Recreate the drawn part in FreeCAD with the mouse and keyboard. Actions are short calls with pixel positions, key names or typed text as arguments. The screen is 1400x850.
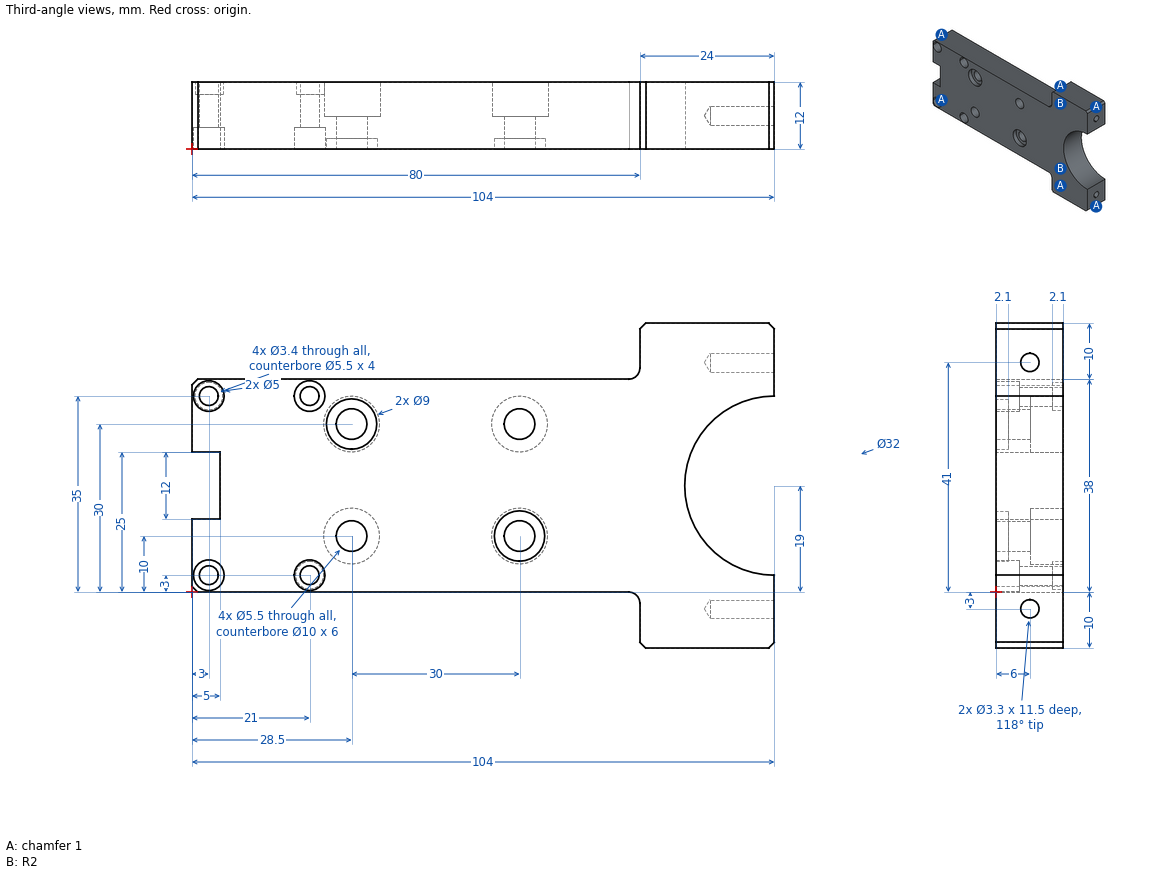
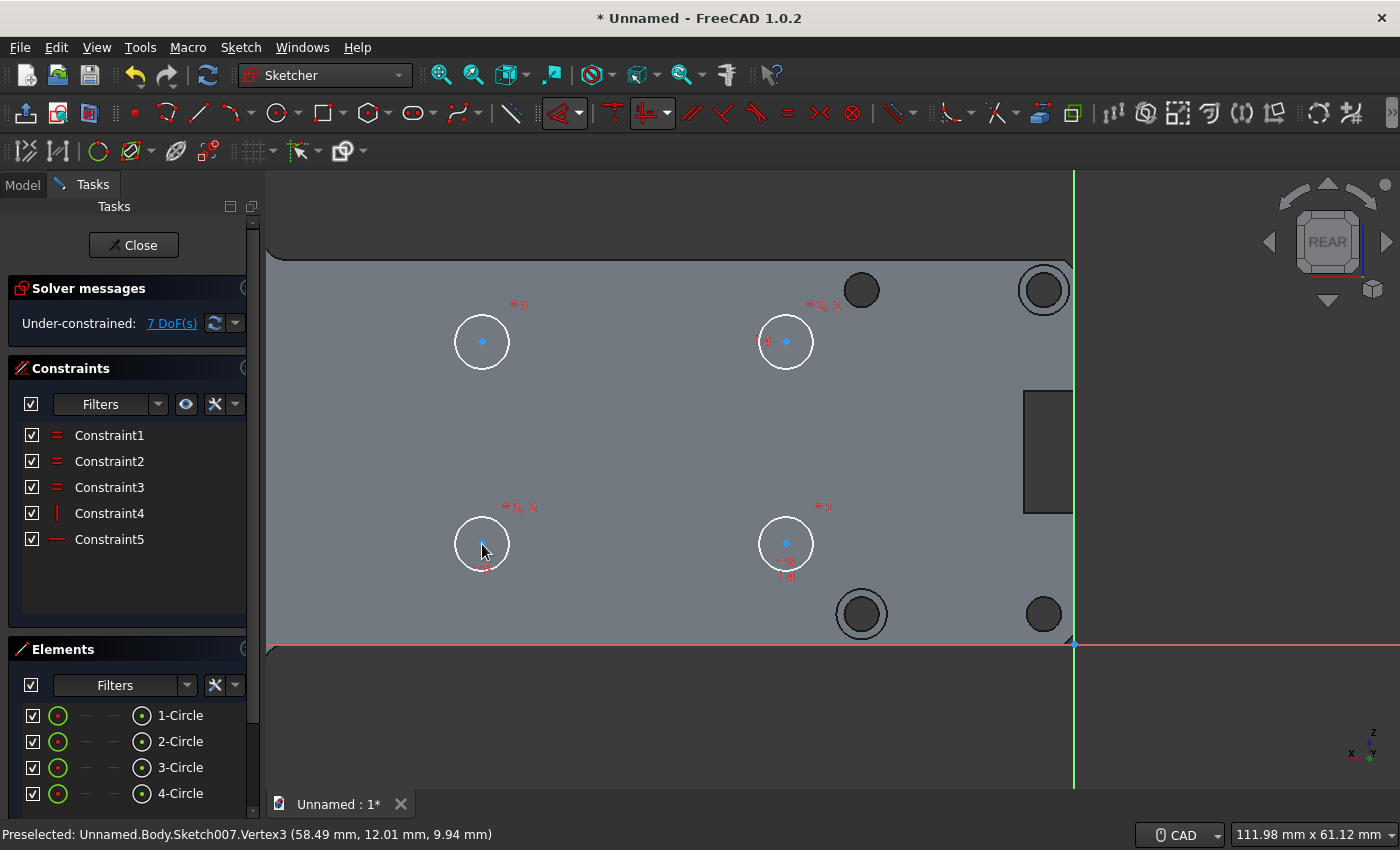
click(482, 544)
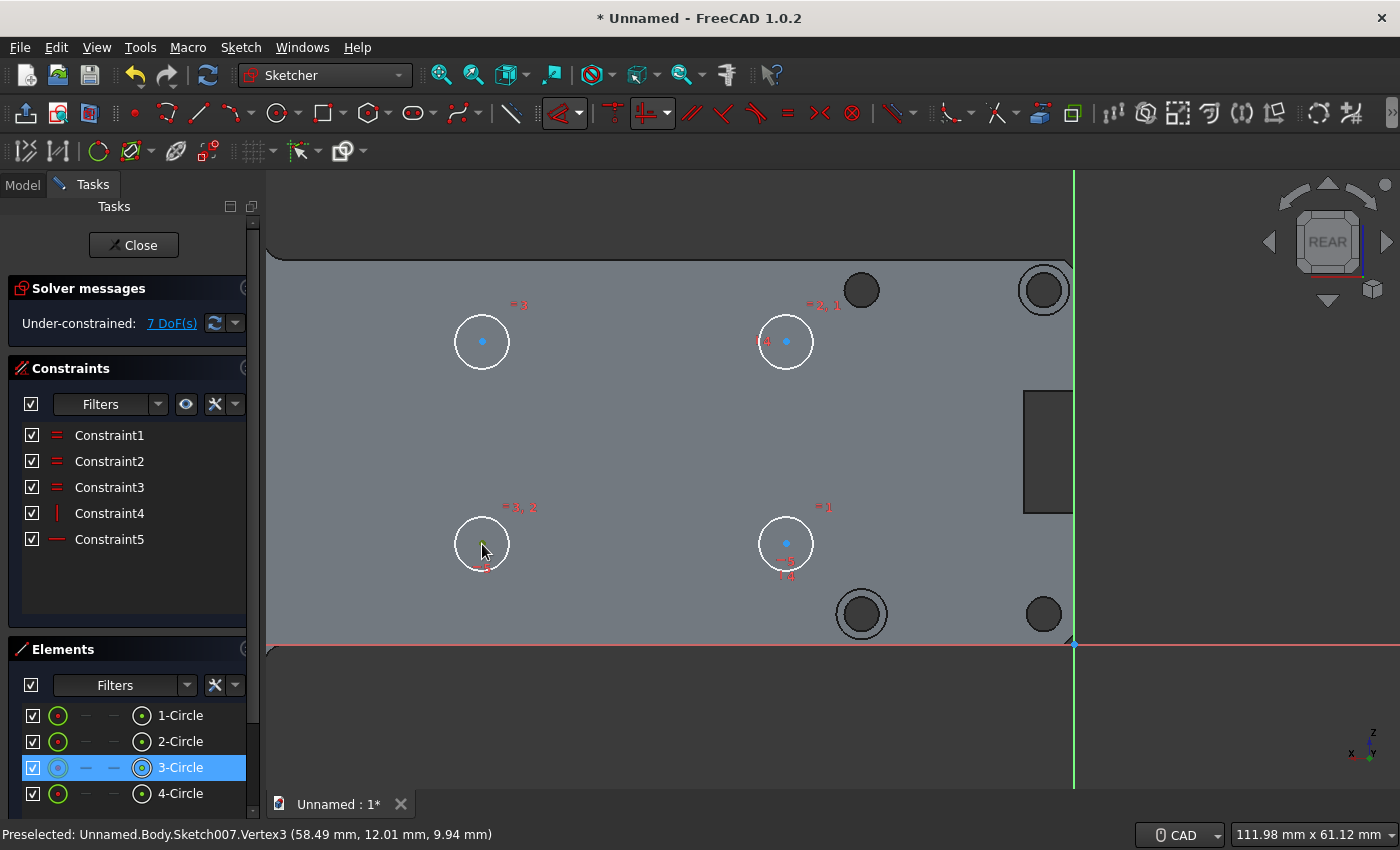
click(482, 342)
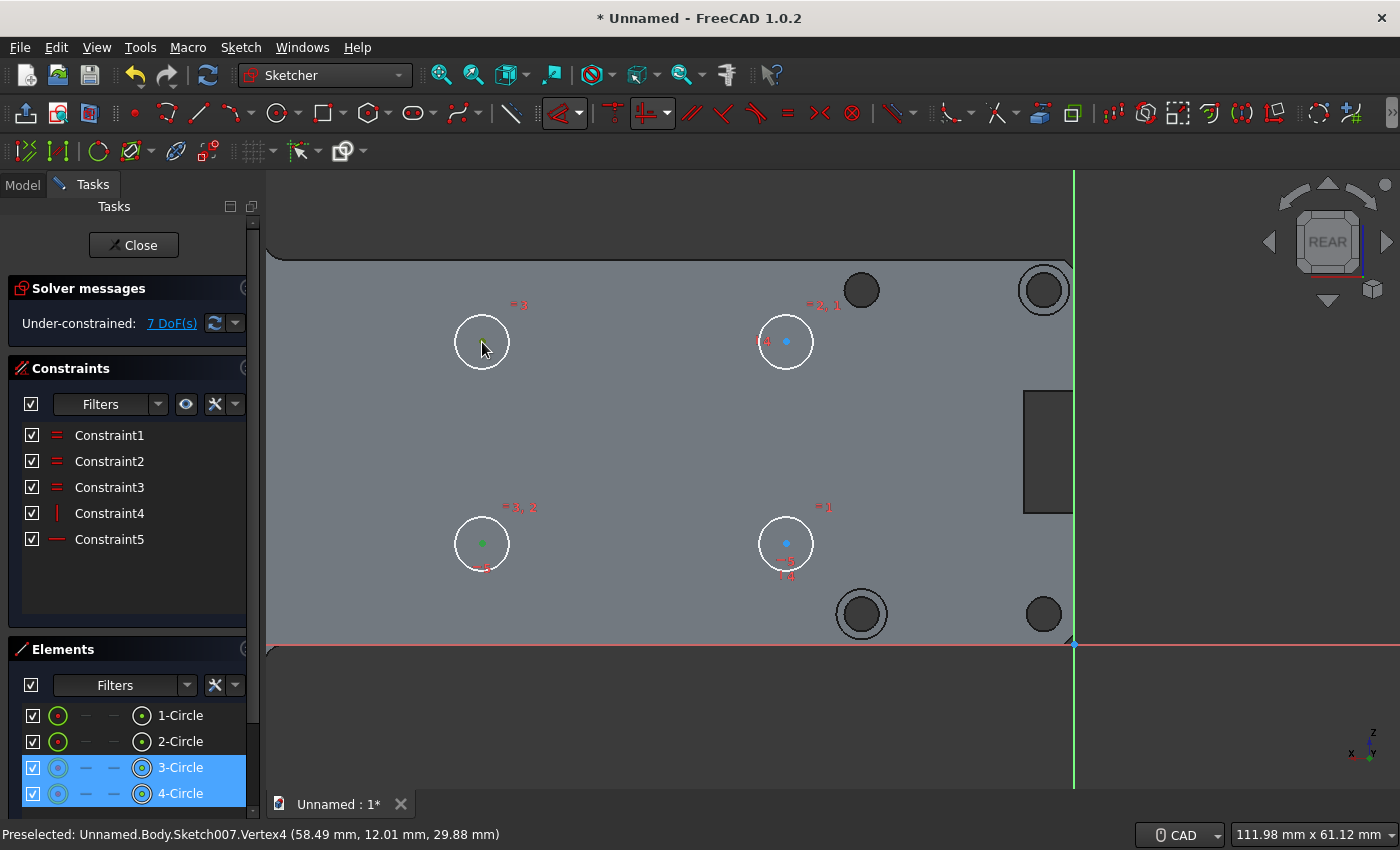
key(v)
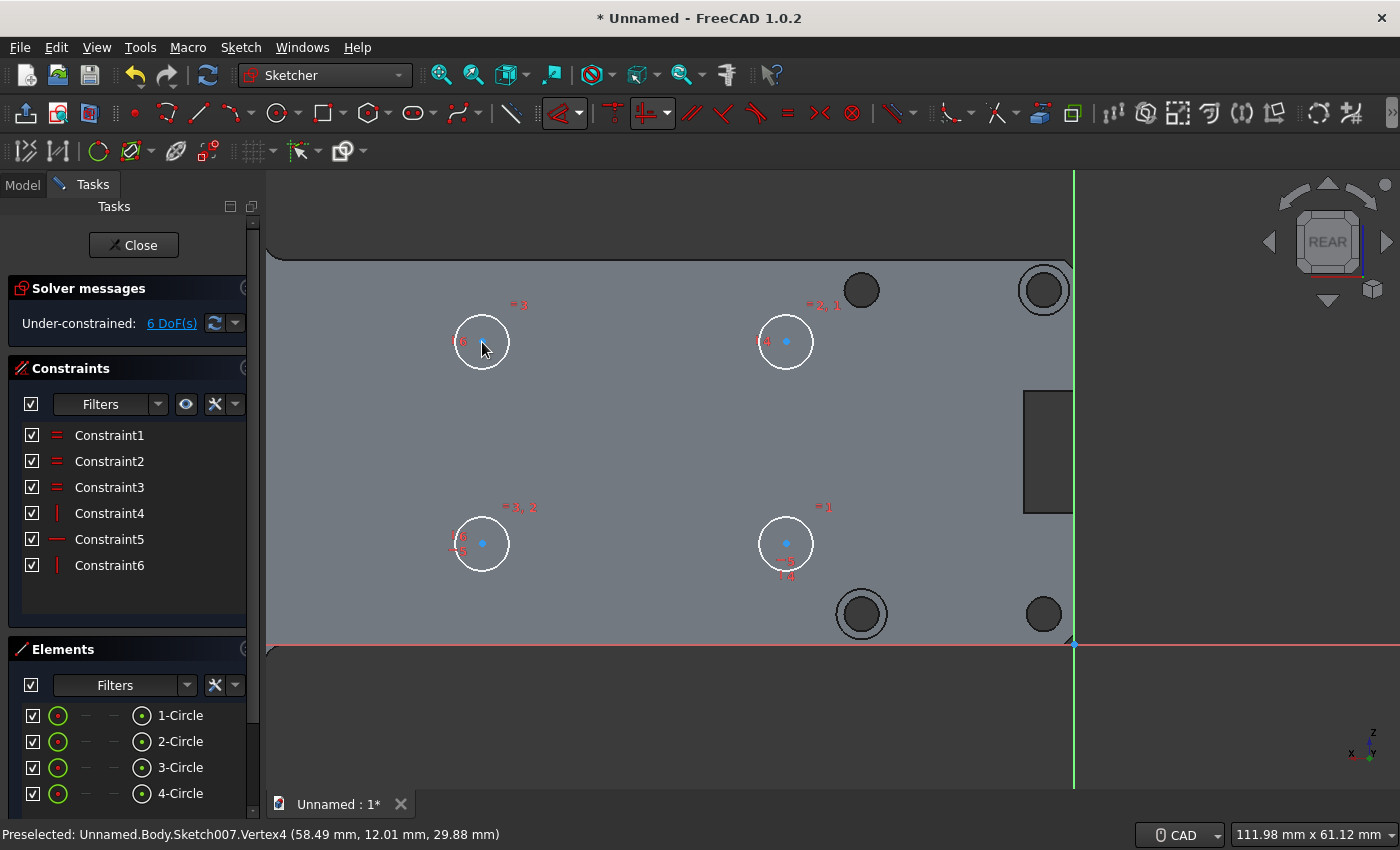
click(786, 342)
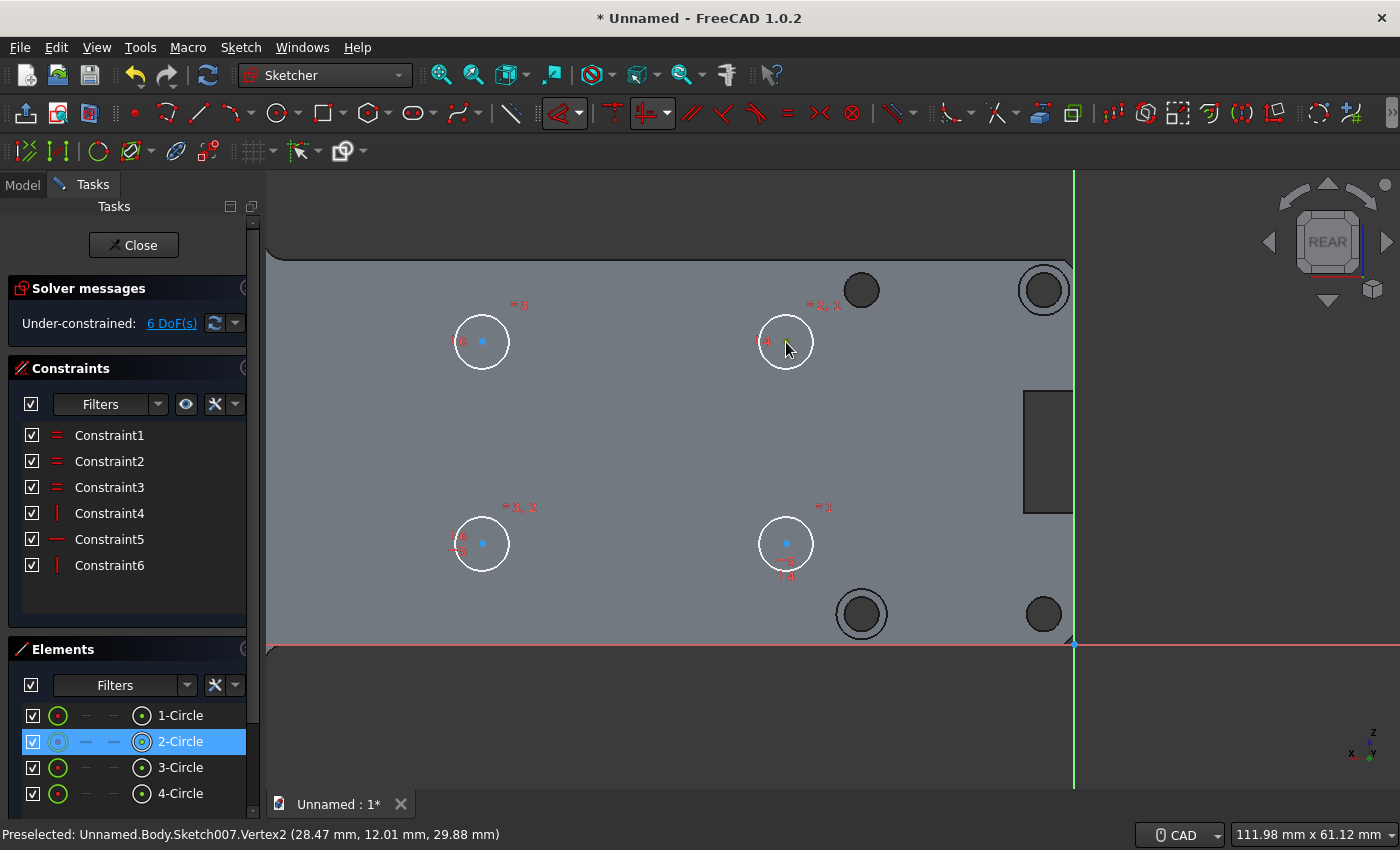
click(482, 342)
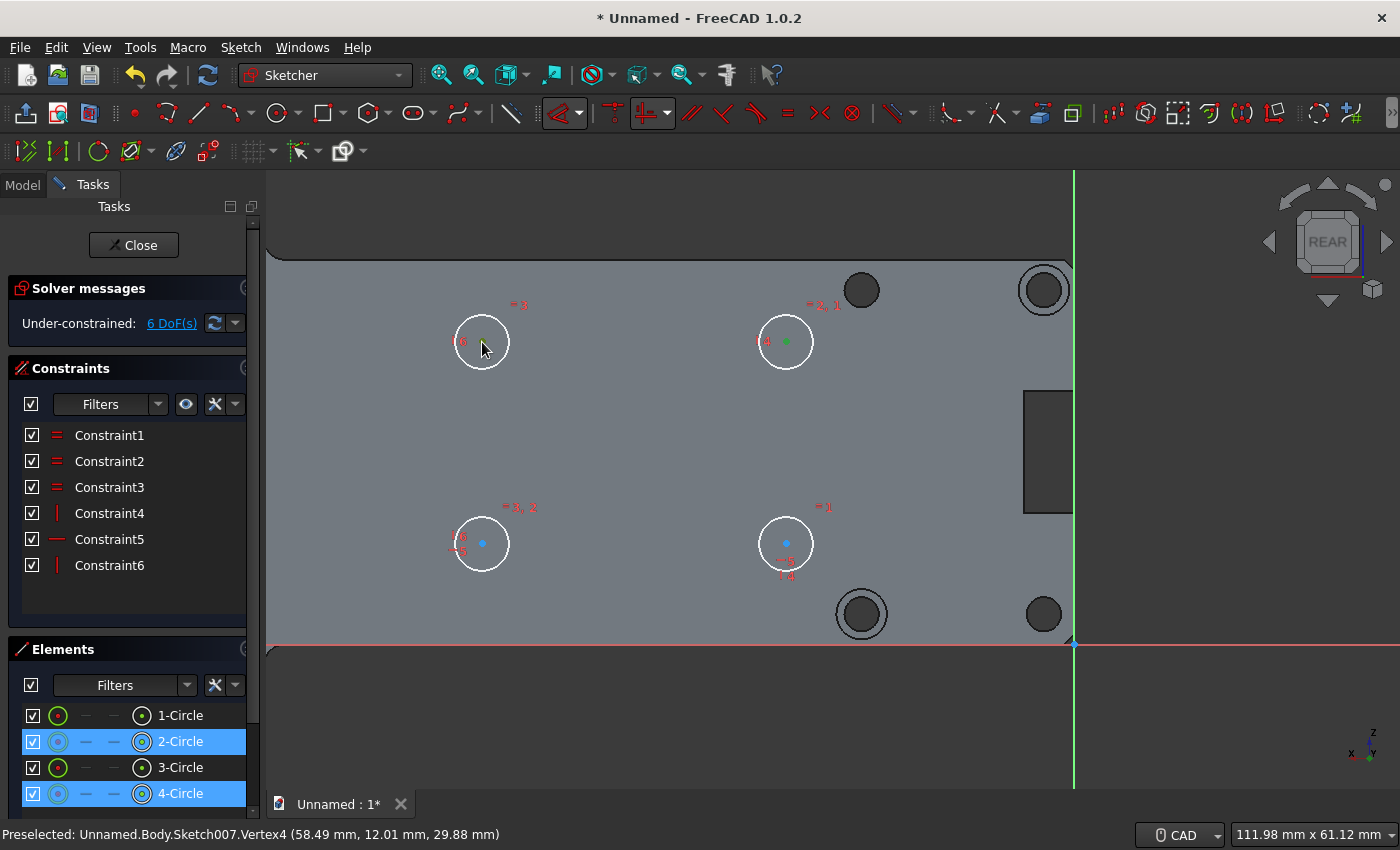
key(h)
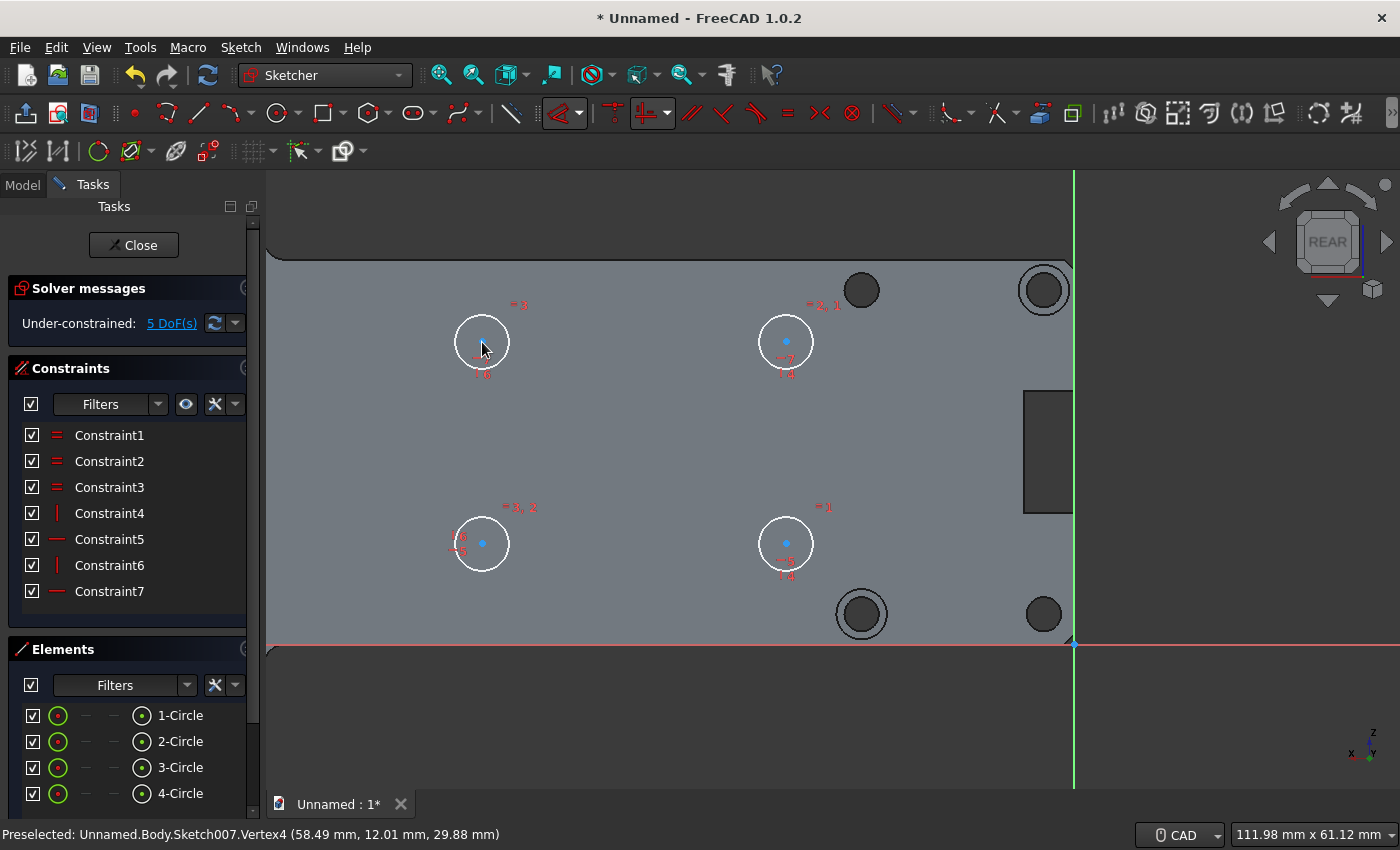
click(805, 525)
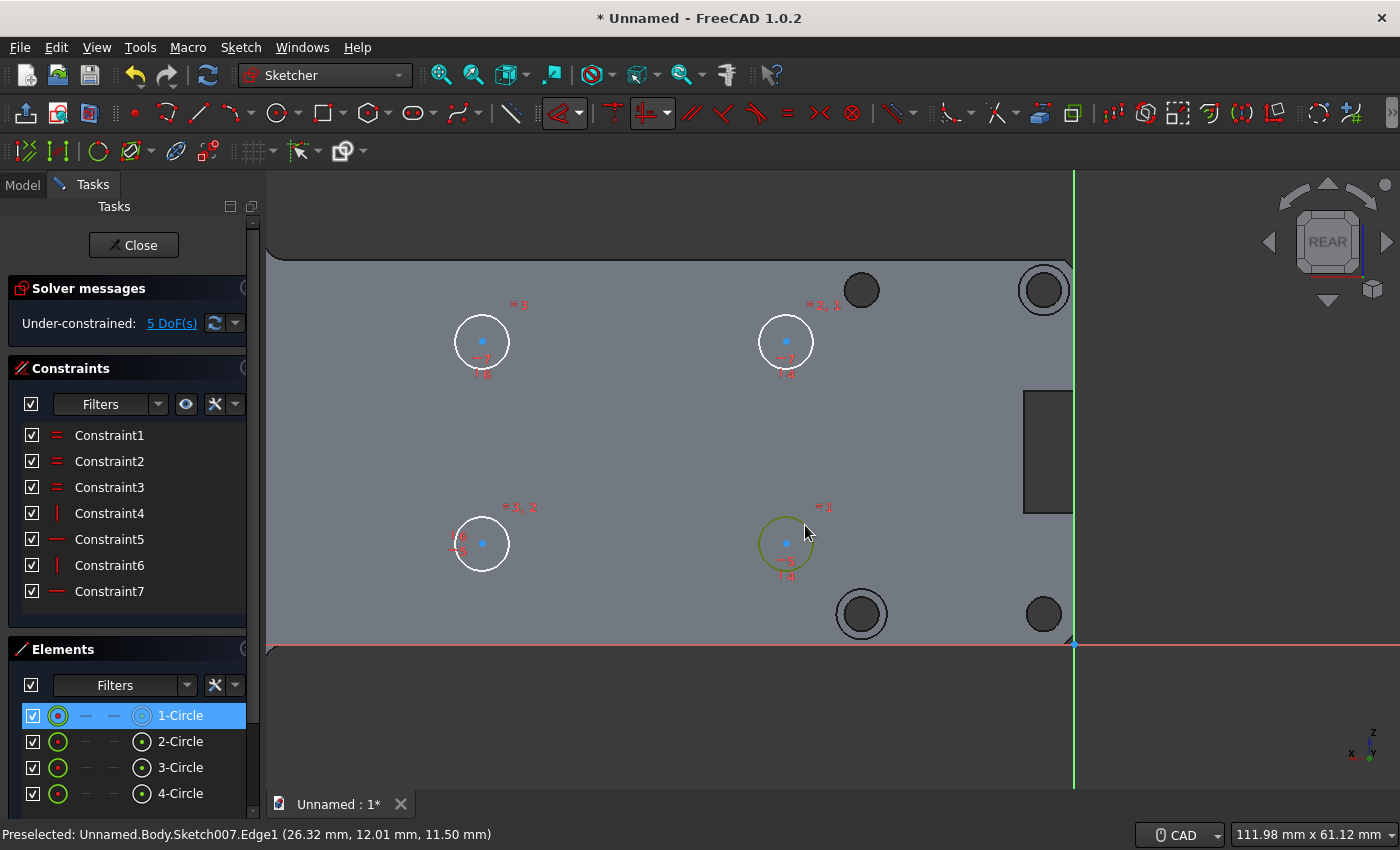
key(k)
key(o)